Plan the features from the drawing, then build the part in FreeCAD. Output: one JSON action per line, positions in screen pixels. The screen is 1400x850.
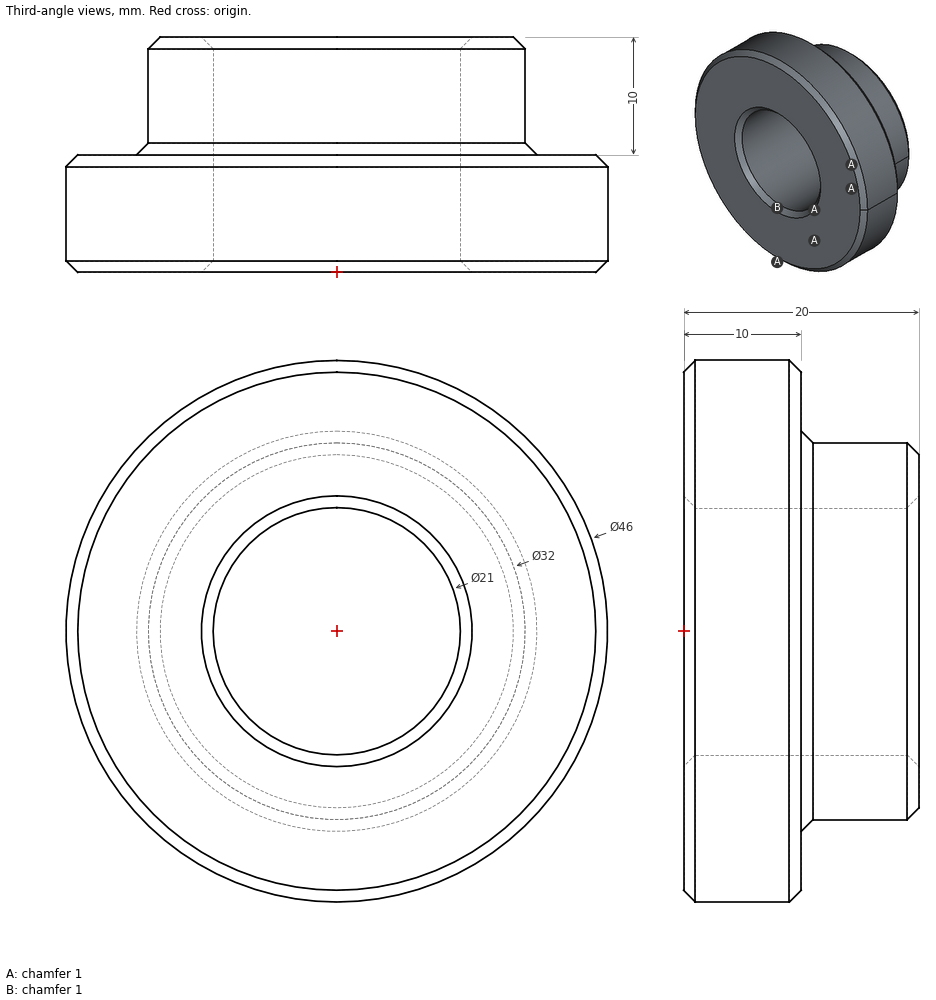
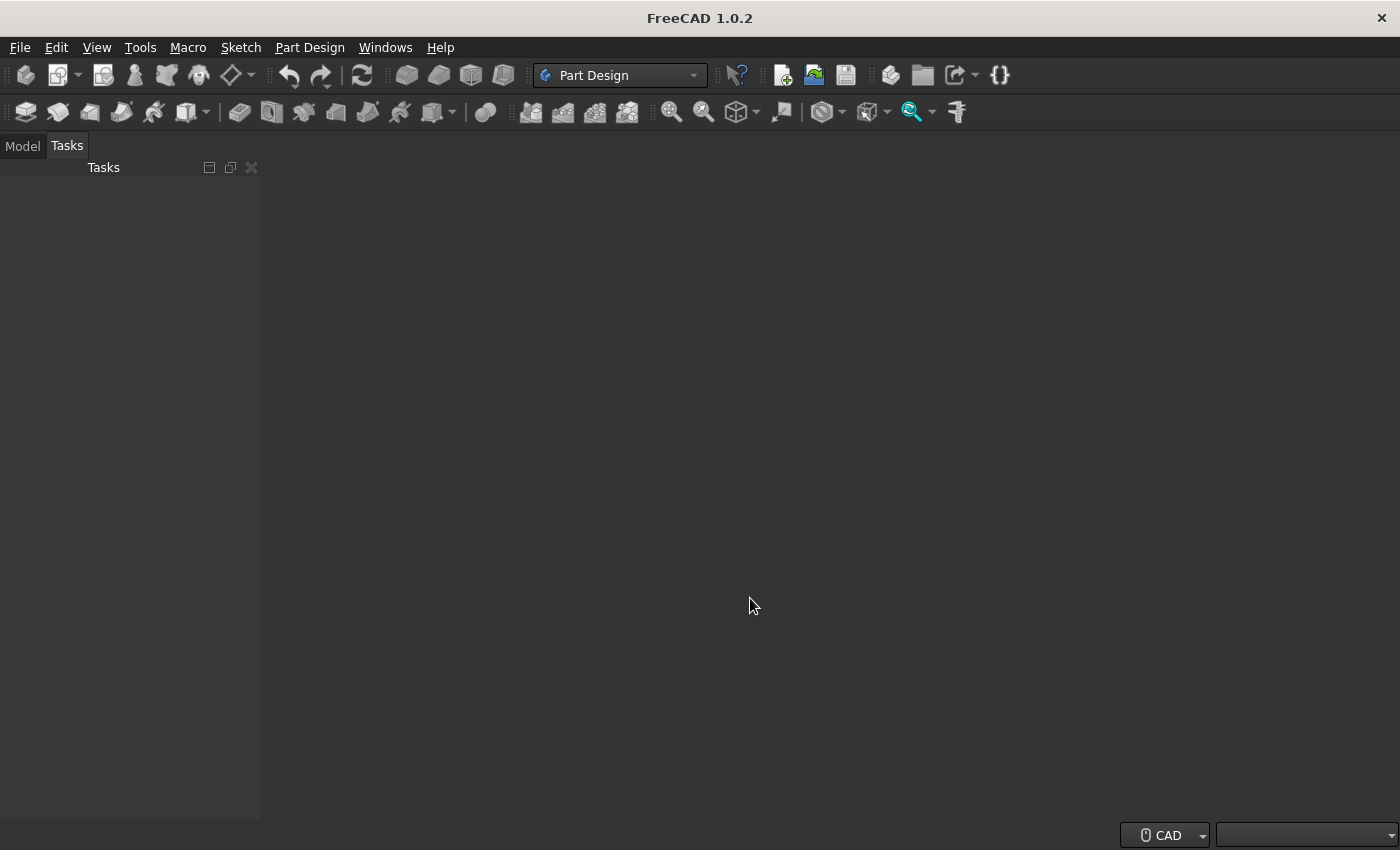
{"action": "left_click", "coordinate": [782, 76]}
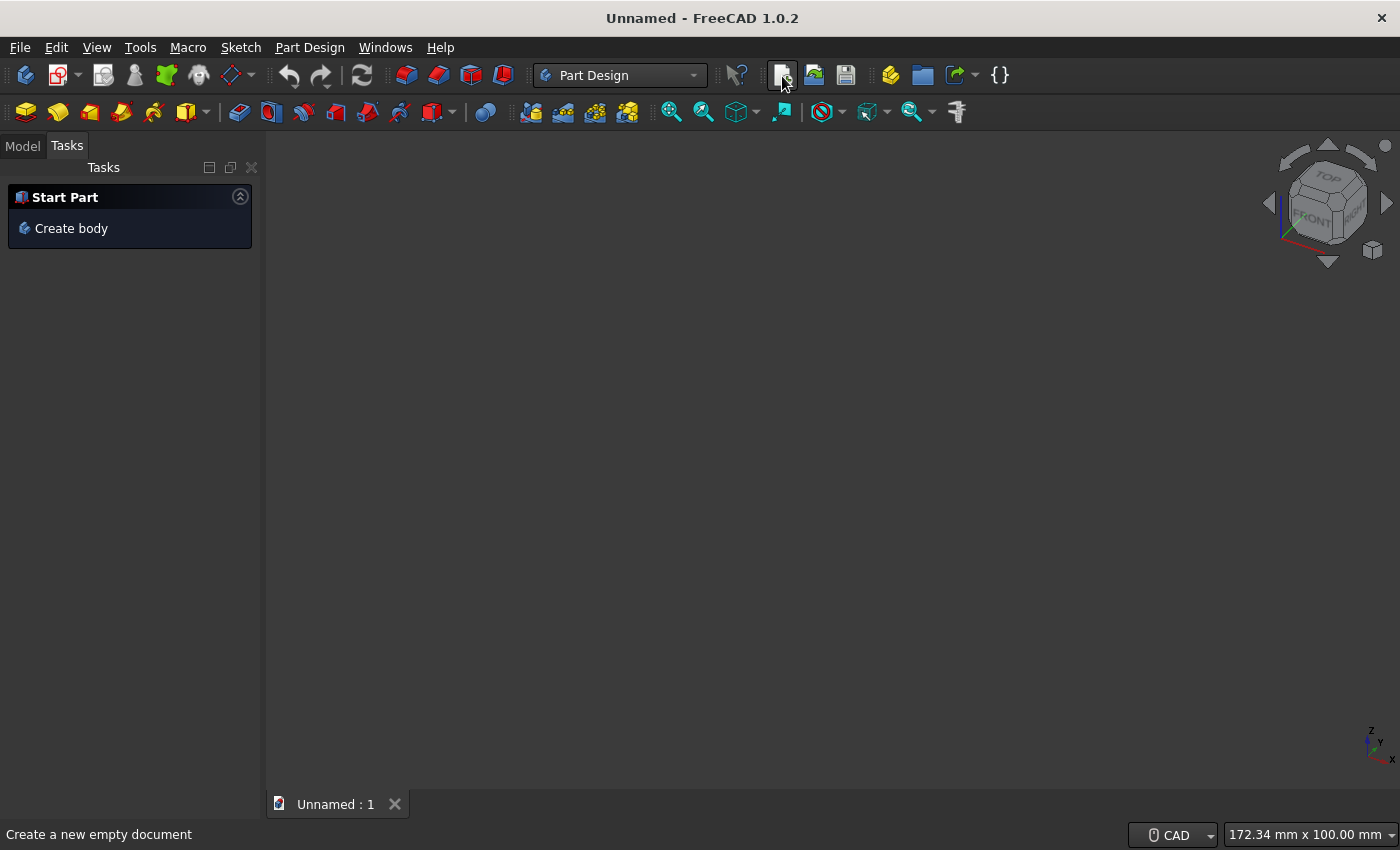
{"action": "left_click", "coordinate": [58, 76]}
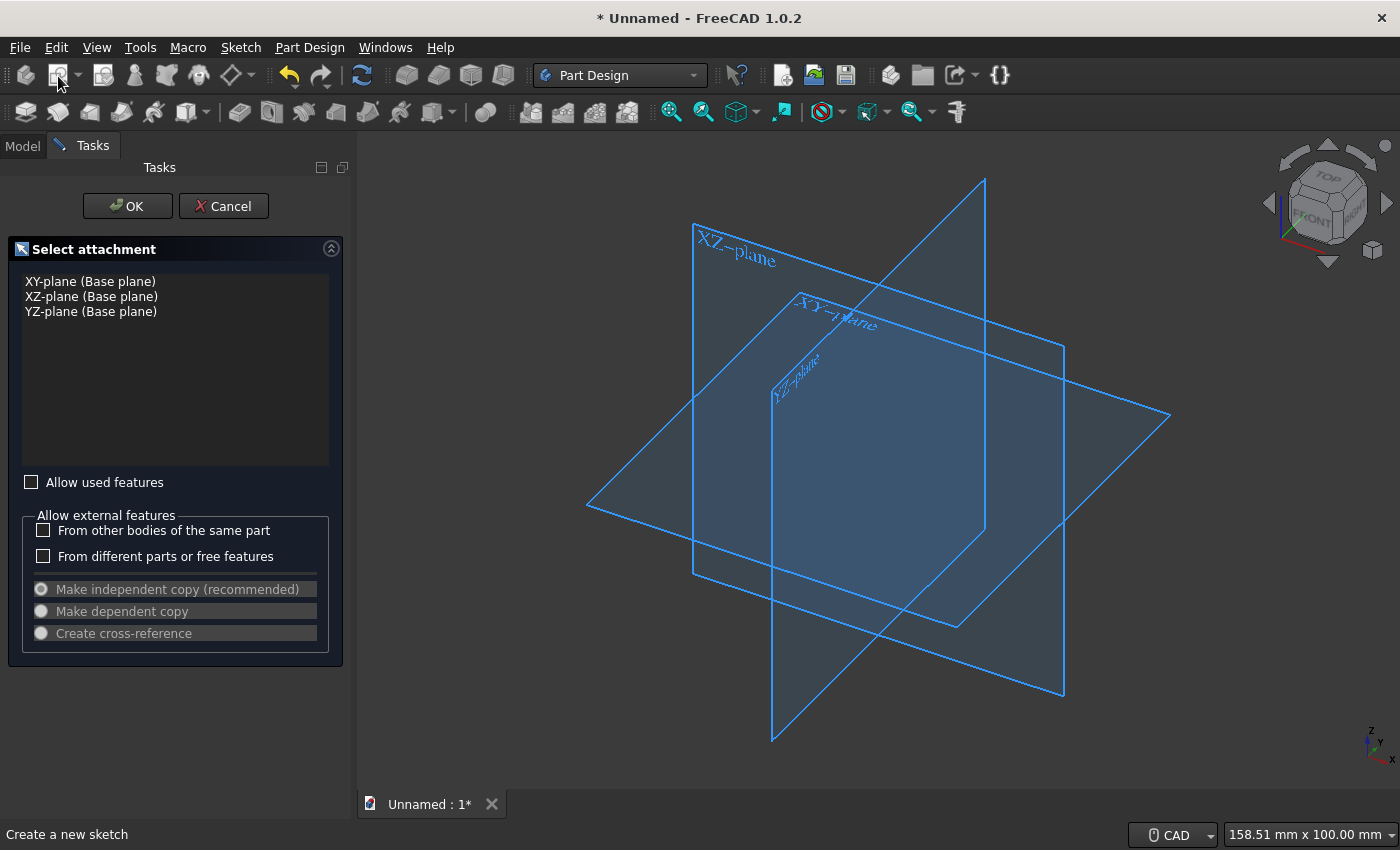
{"action": "left_click", "coordinate": [82, 296]}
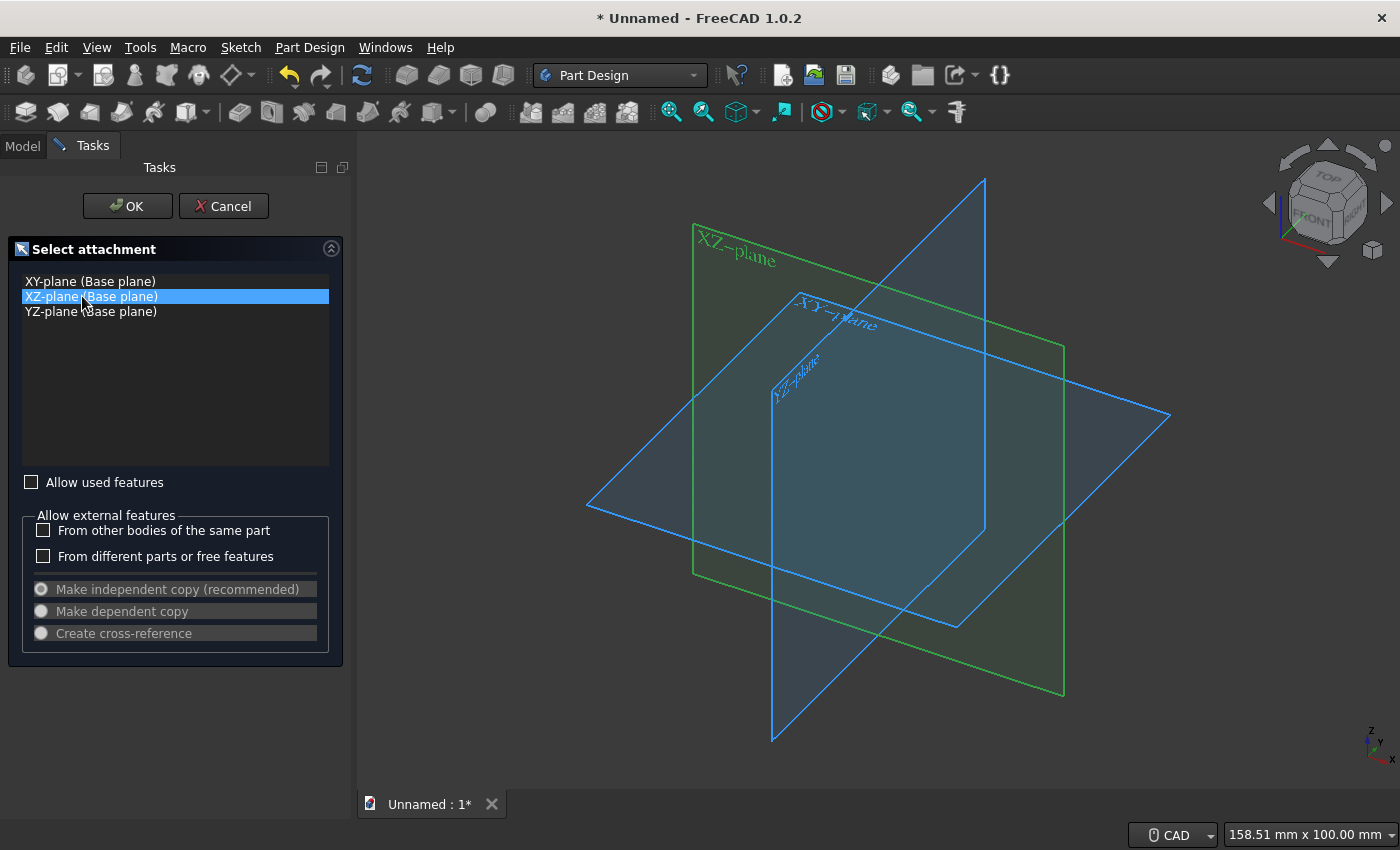
{"action": "left_click", "coordinate": [128, 206]}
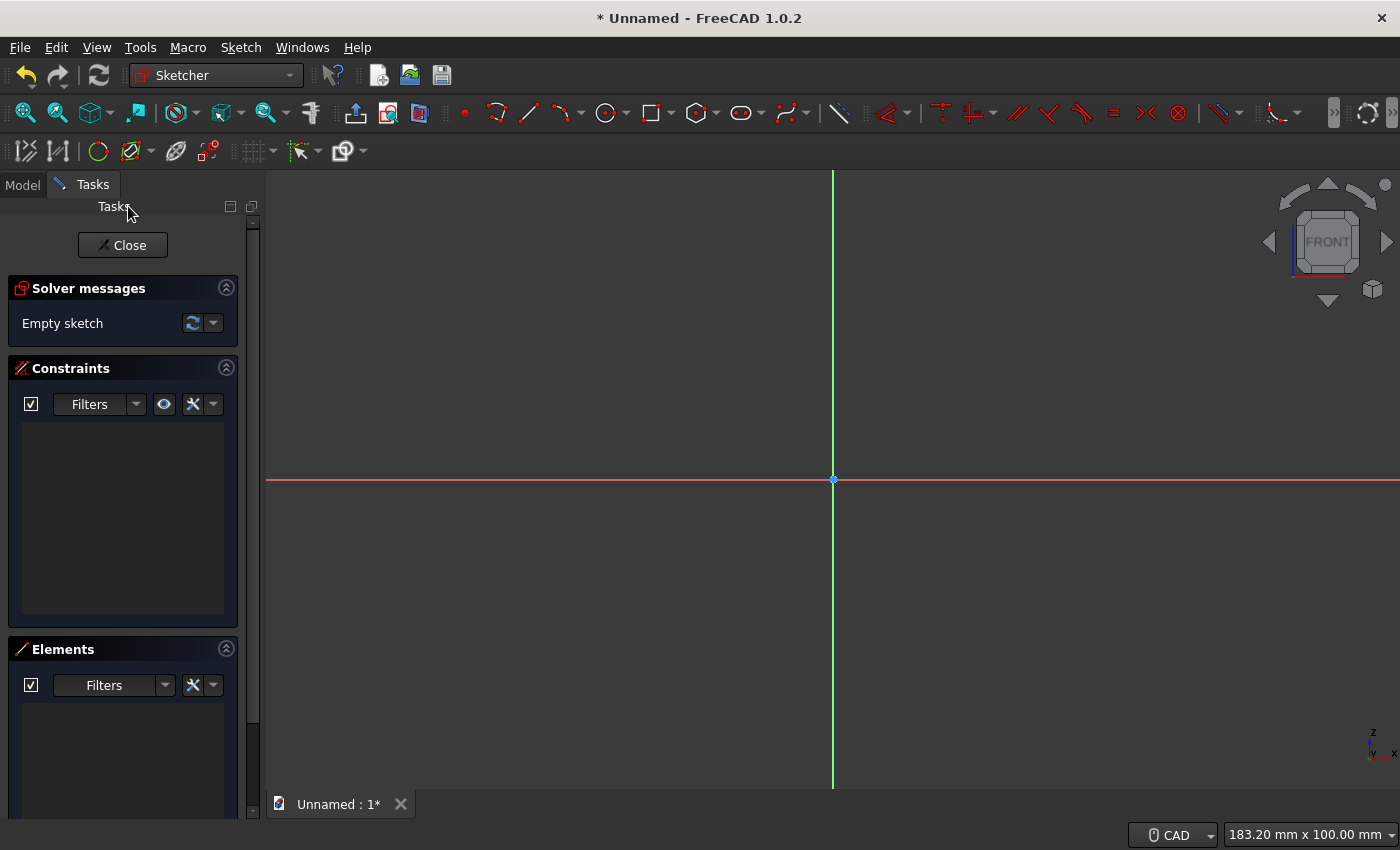
{"action": "scroll", "coordinate": [972, 480], "scroll_direction": "up", "scroll_amount": 2}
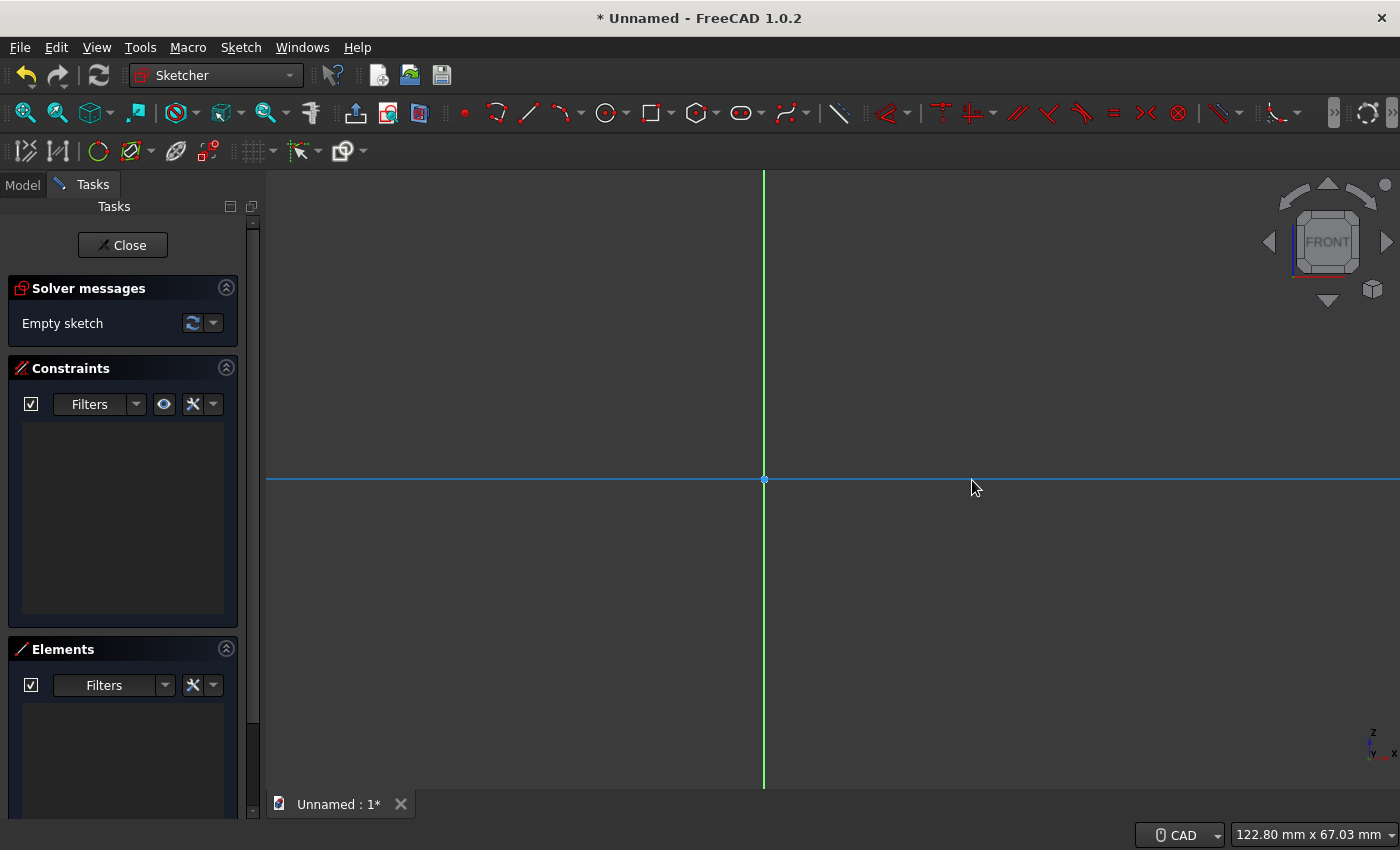
{"action": "key", "text": "g c"}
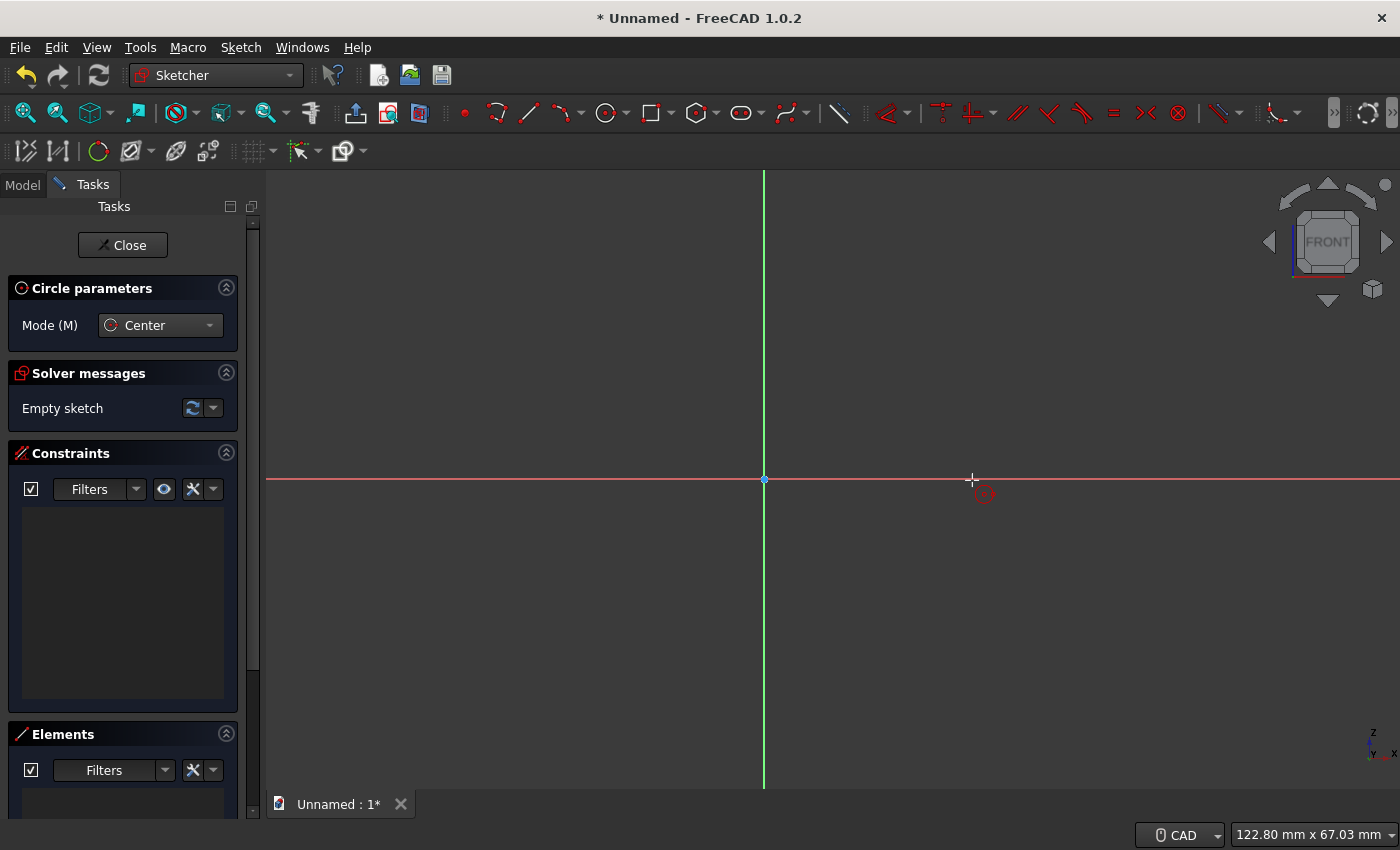
{"action": "left_click", "coordinate": [764, 479]}
{"action": "left_click", "coordinate": [915, 329]}
{"action": "key", "text": "Escape"}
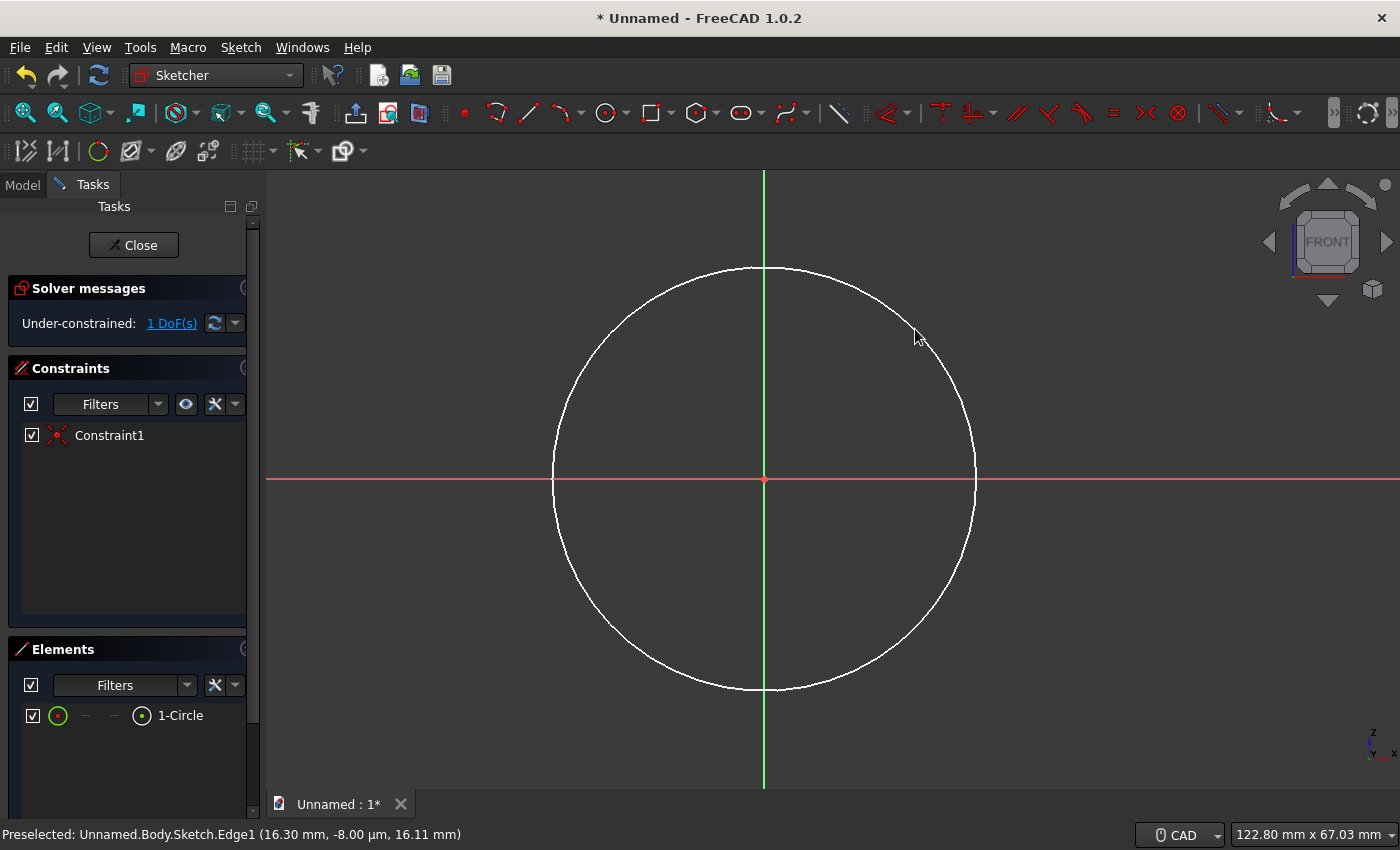
{"action": "key", "text": "d"}